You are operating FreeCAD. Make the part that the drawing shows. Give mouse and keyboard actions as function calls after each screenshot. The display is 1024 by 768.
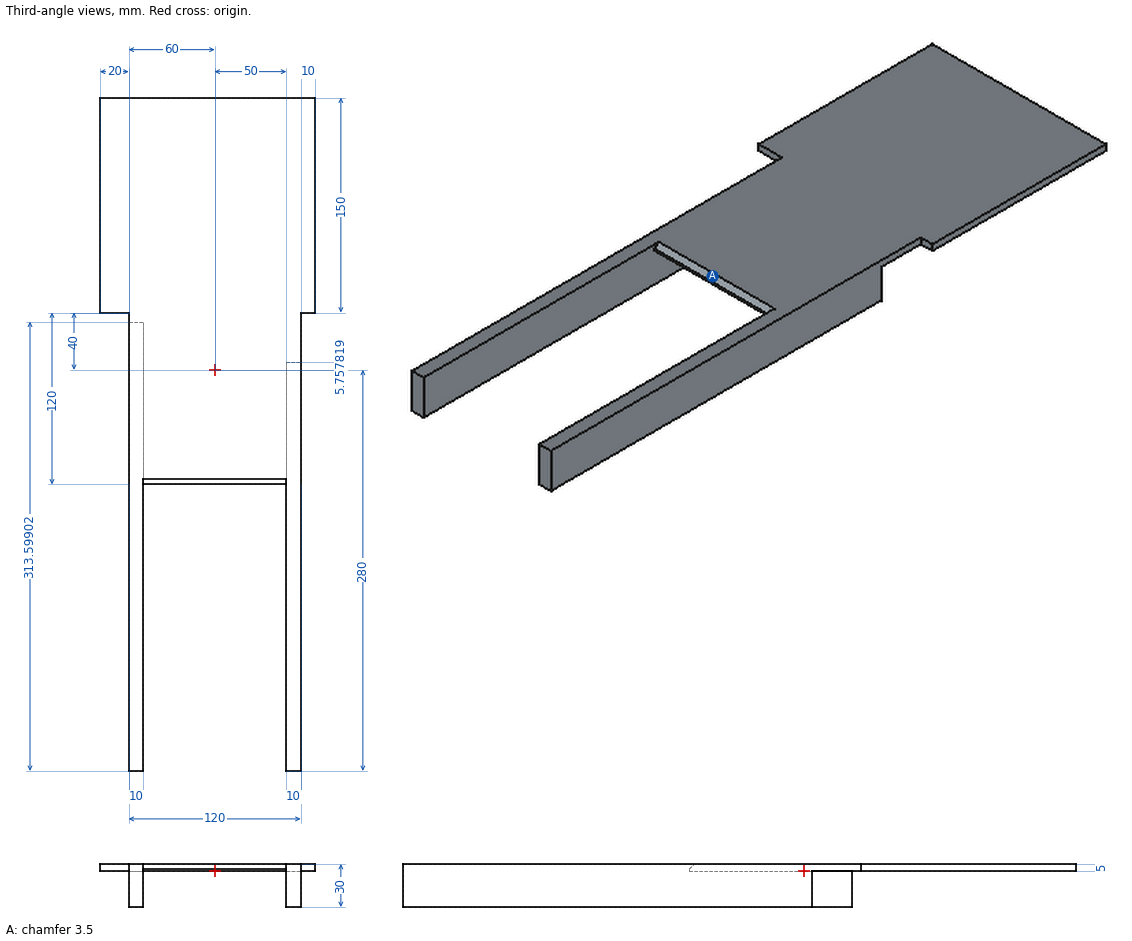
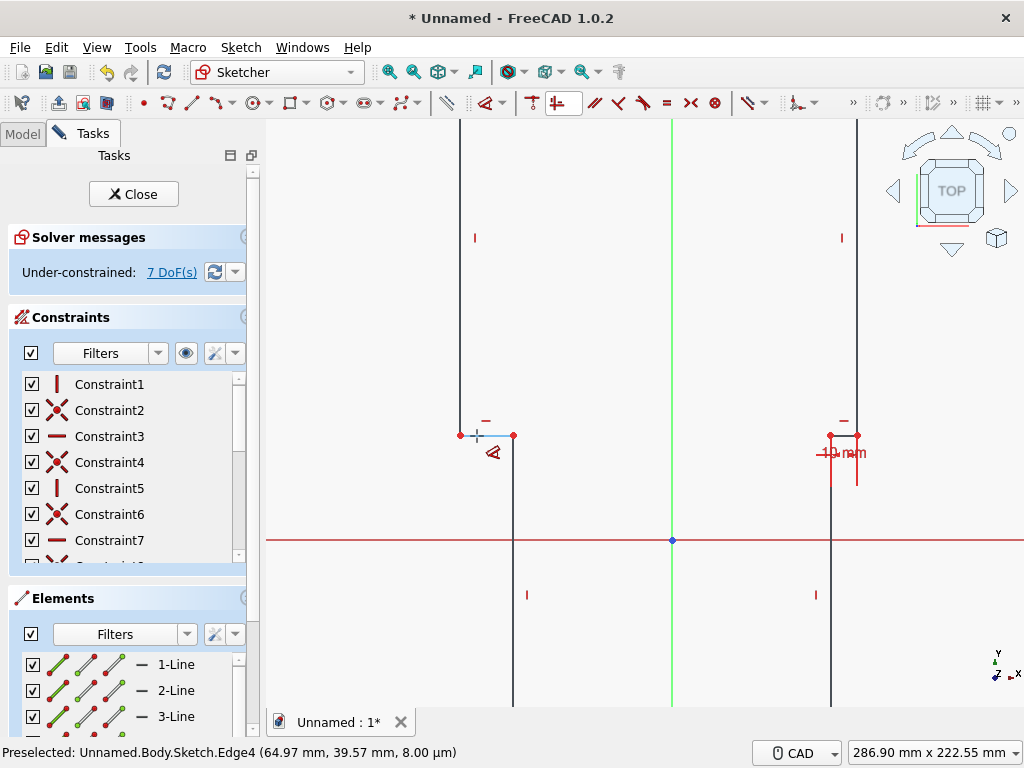
click(476, 436)
click(487, 470)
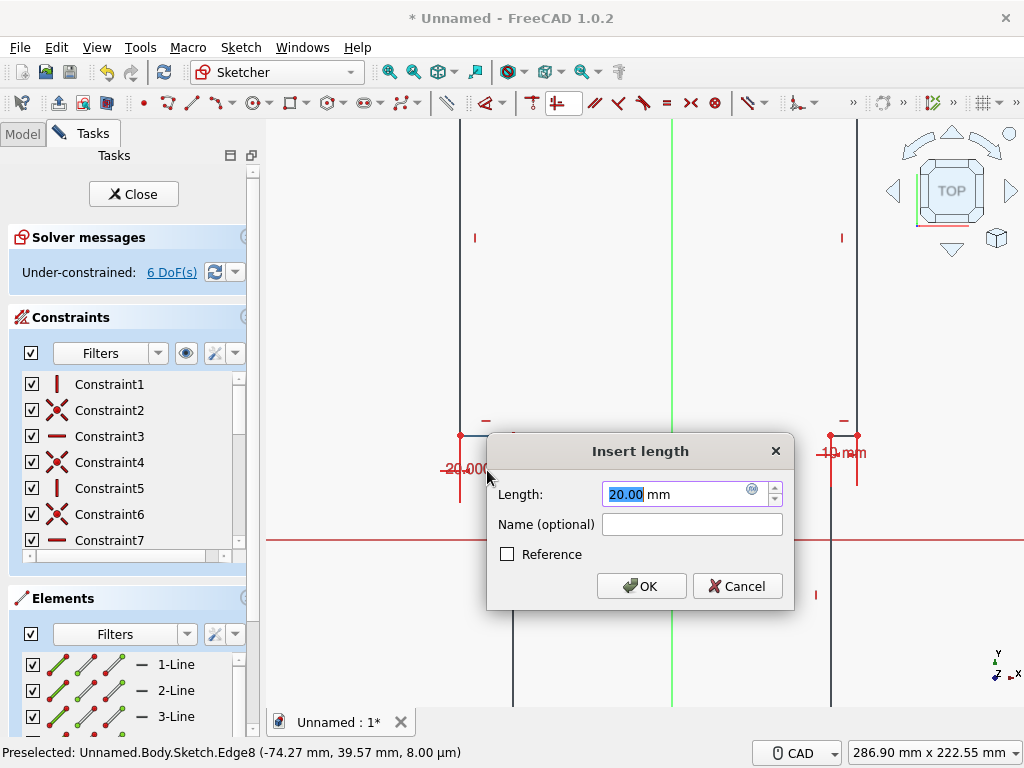
text(20)
key(Return)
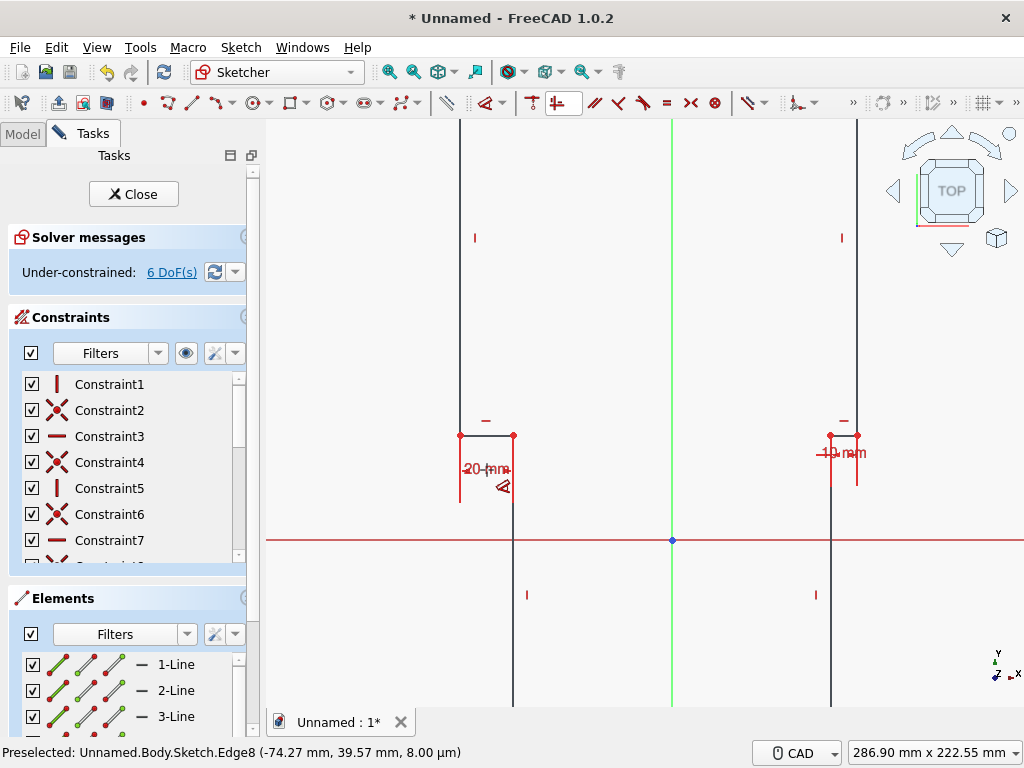
scroll(513, 531, up, 2)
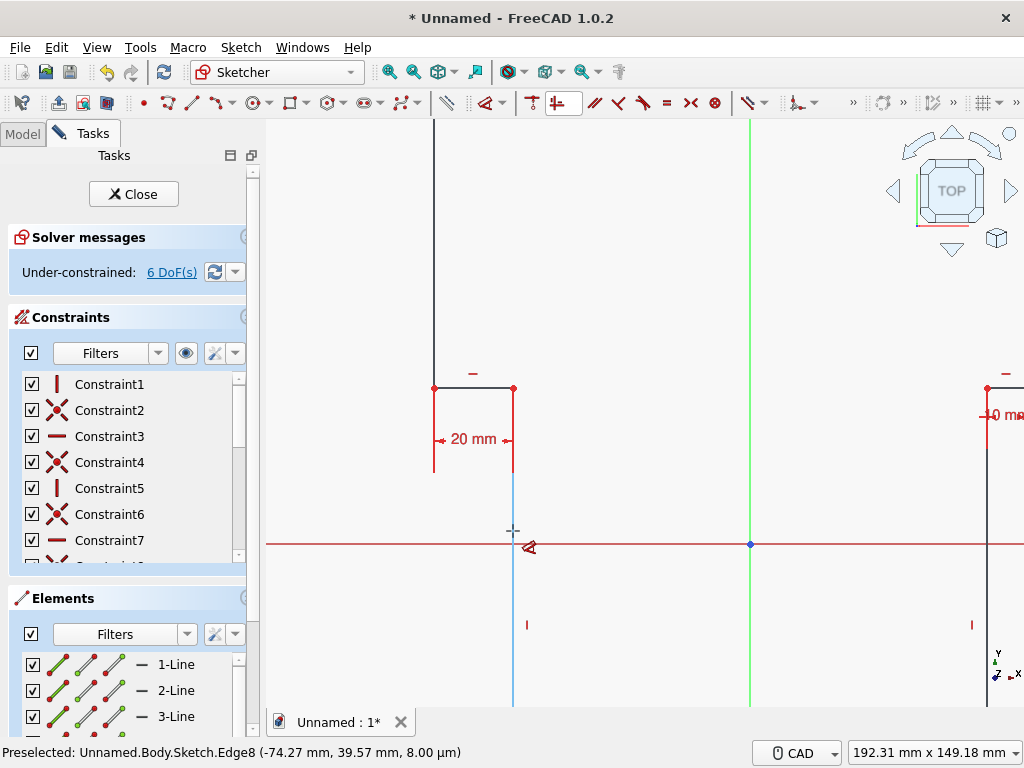
click(513, 530)
click(479, 467)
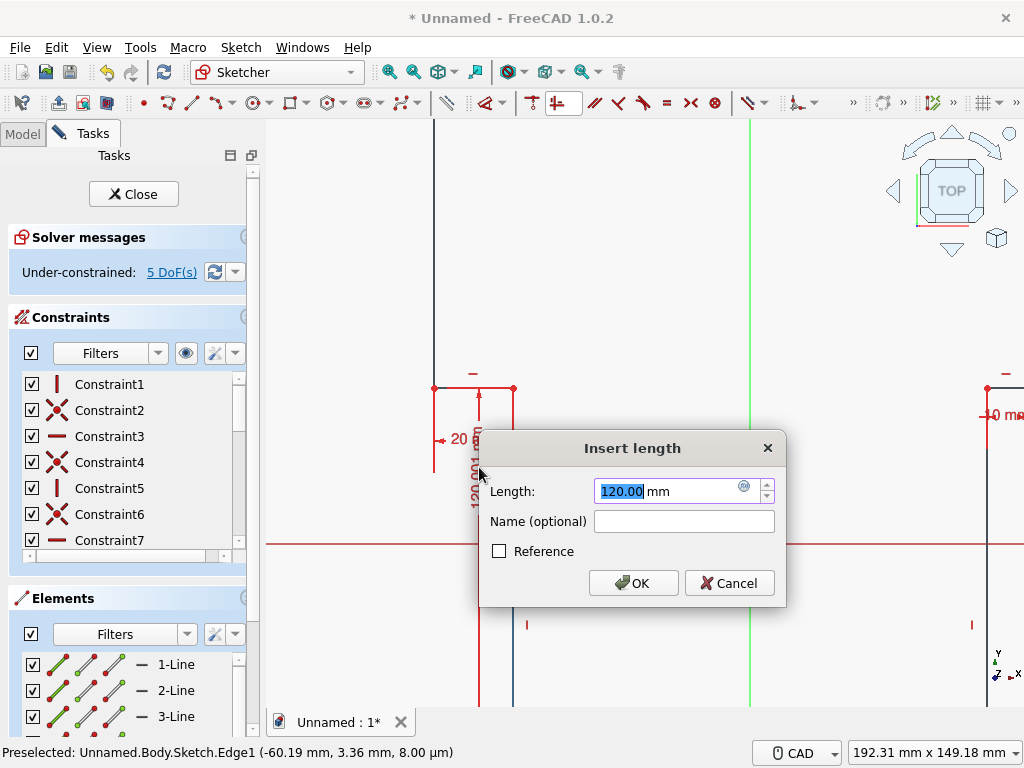
text(120)
key(Return)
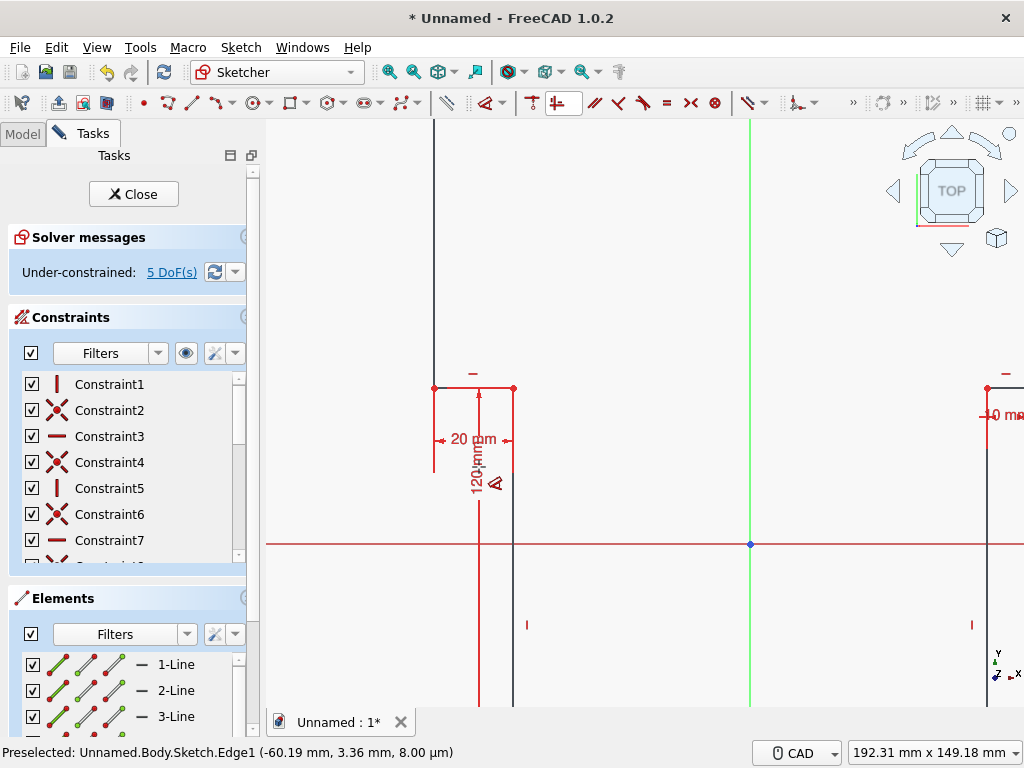
scroll(487, 463, down, 5)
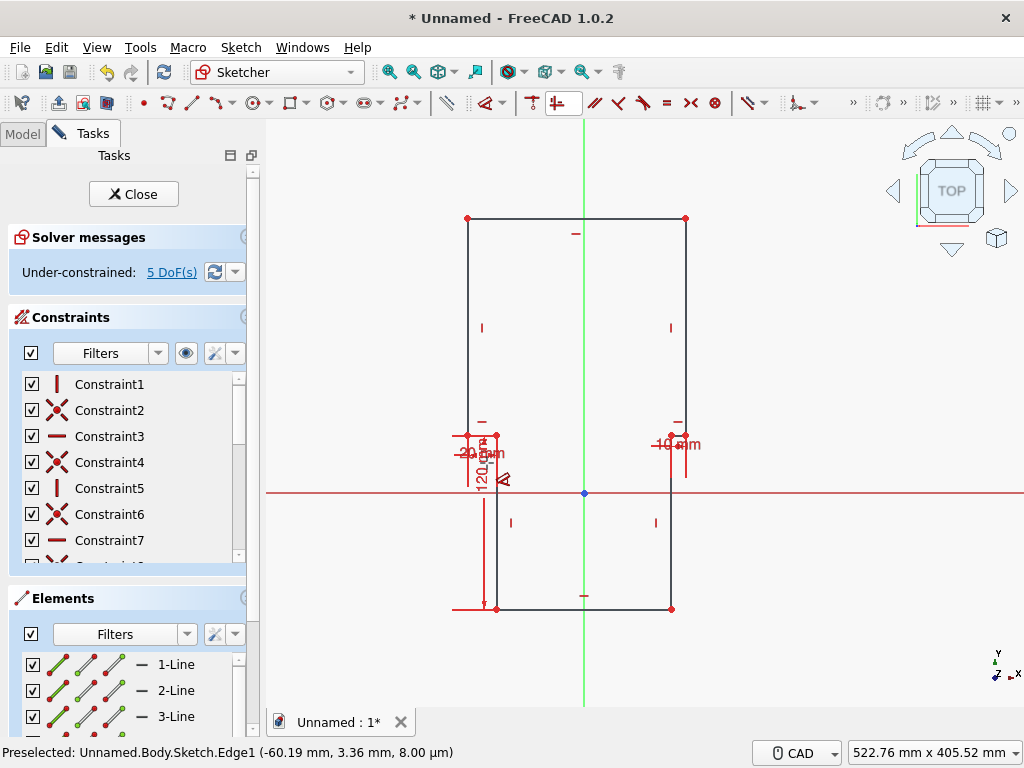
click(549, 610)
click(544, 644)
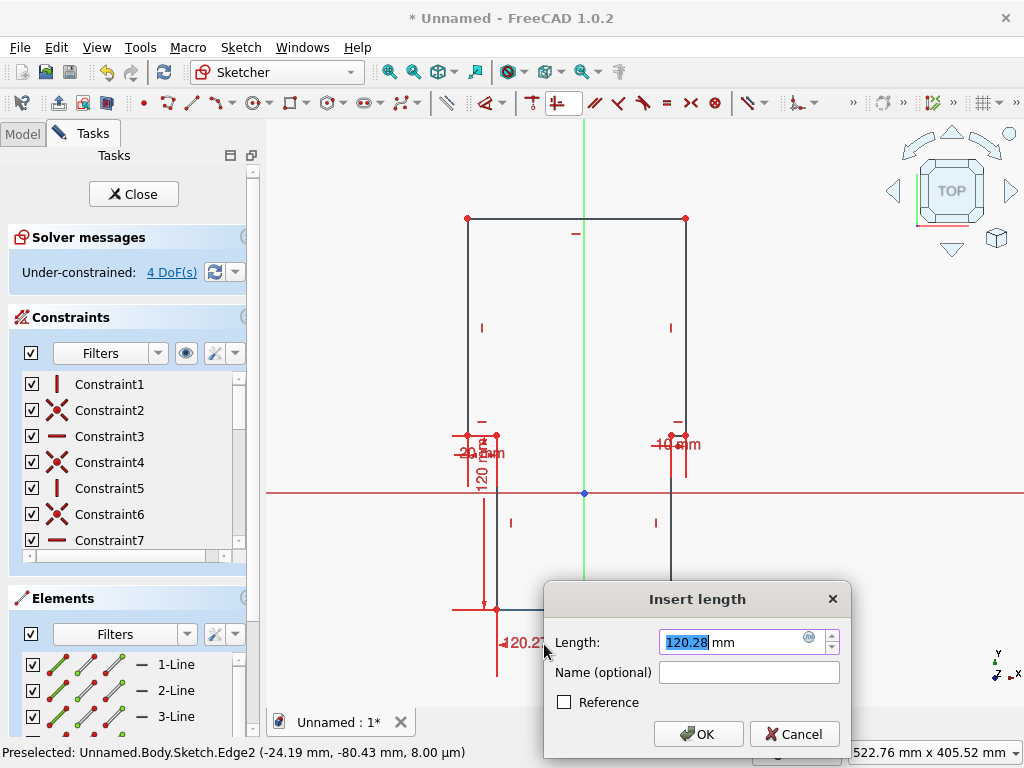
text(120)
key(Return)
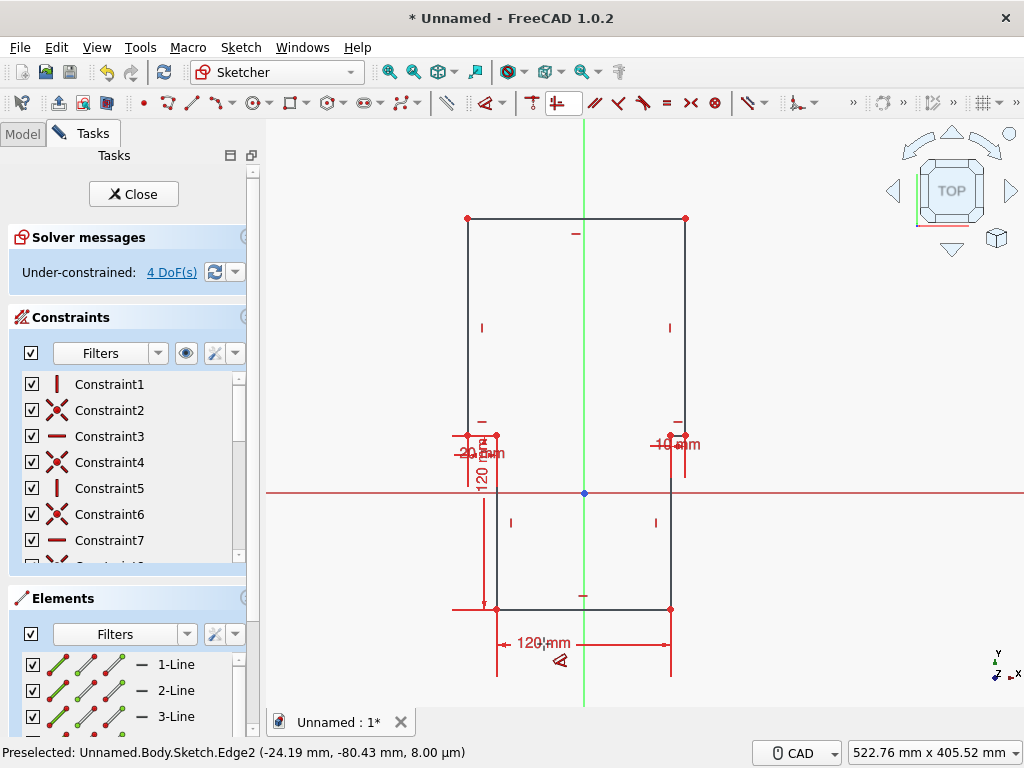
click(671, 558)
click(705, 523)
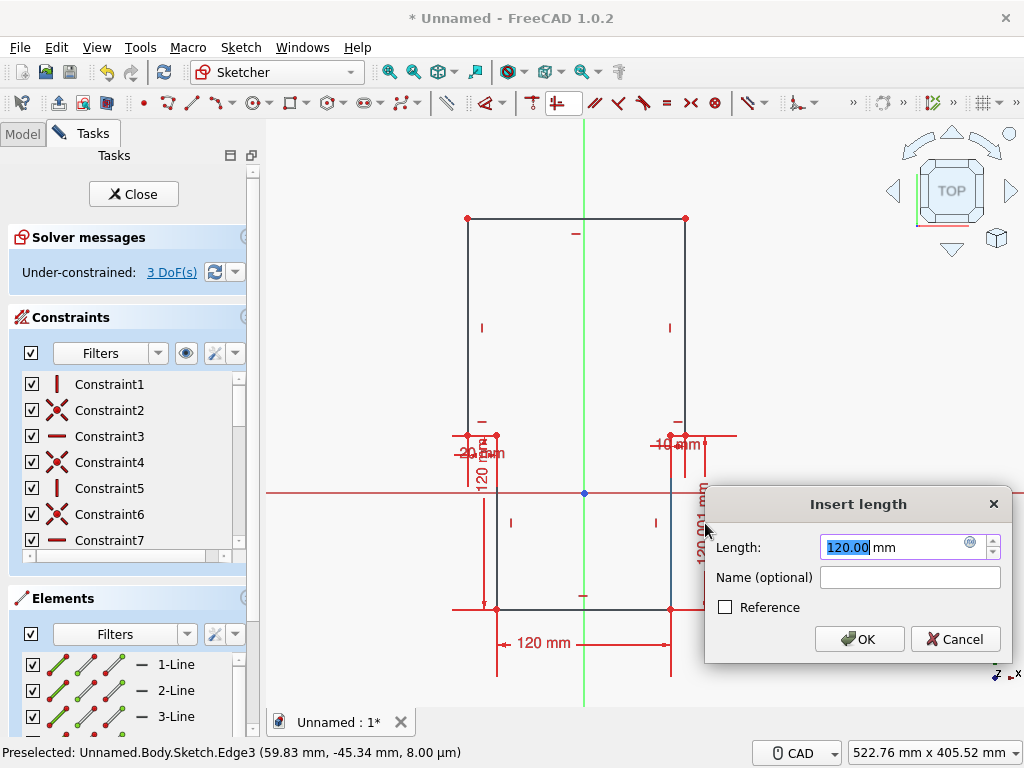
text(120)
key(Return)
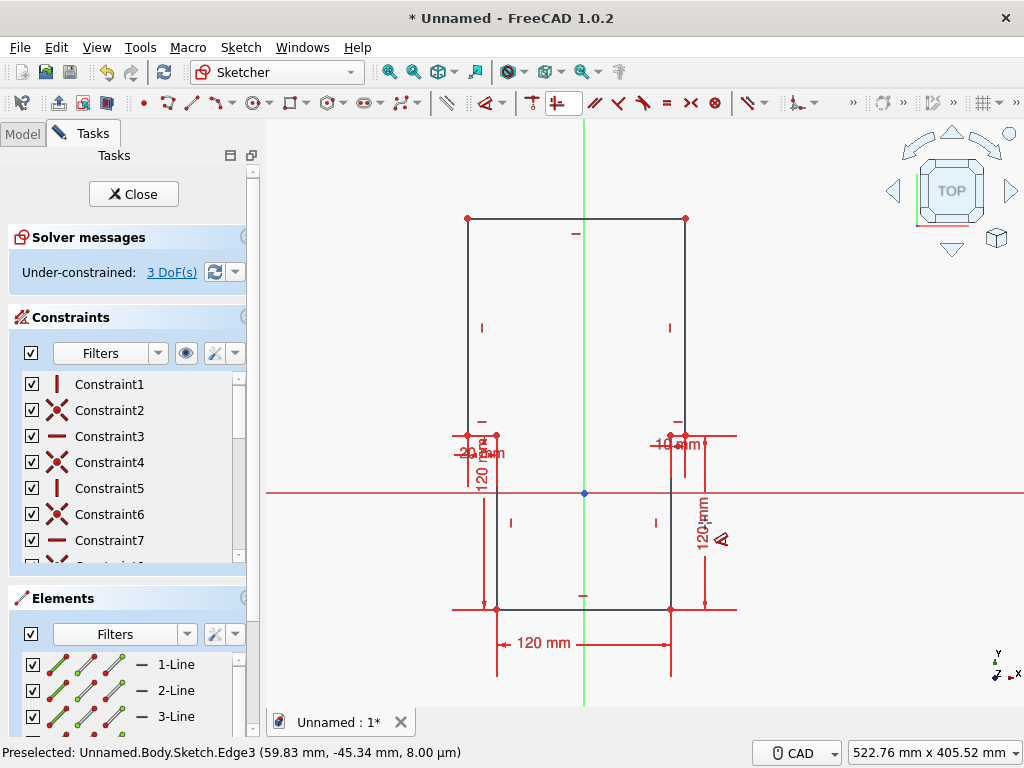
click(685, 371)
click(719, 327)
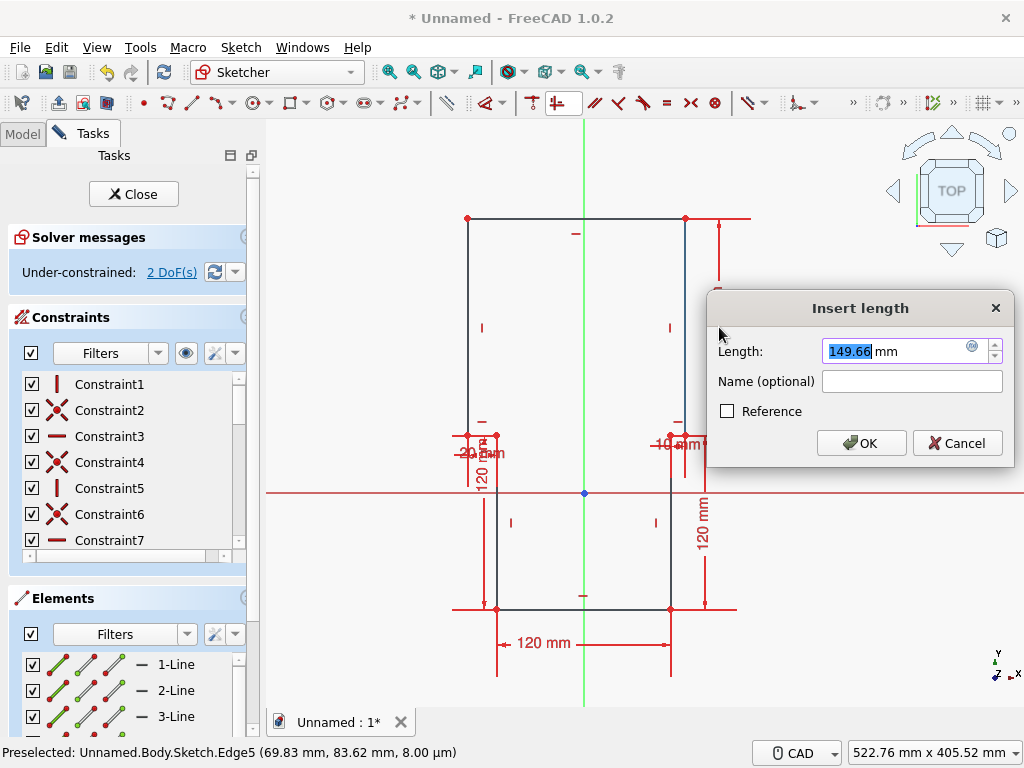
text(150)
key(Return)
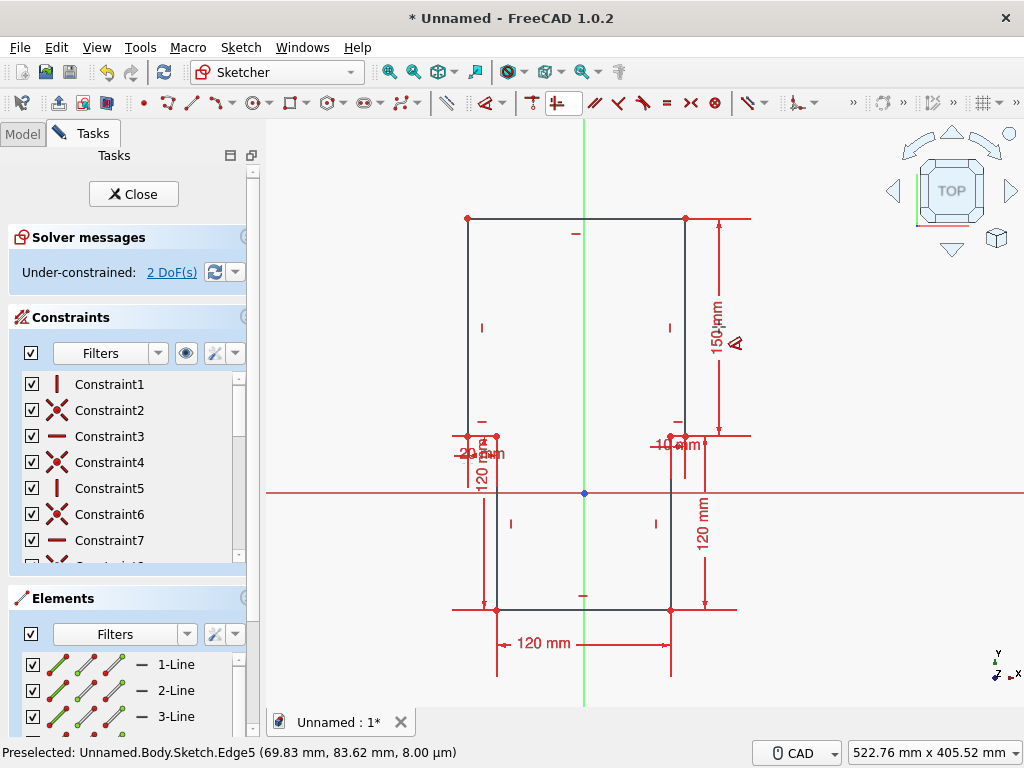
click(497, 436)
click(540, 527)